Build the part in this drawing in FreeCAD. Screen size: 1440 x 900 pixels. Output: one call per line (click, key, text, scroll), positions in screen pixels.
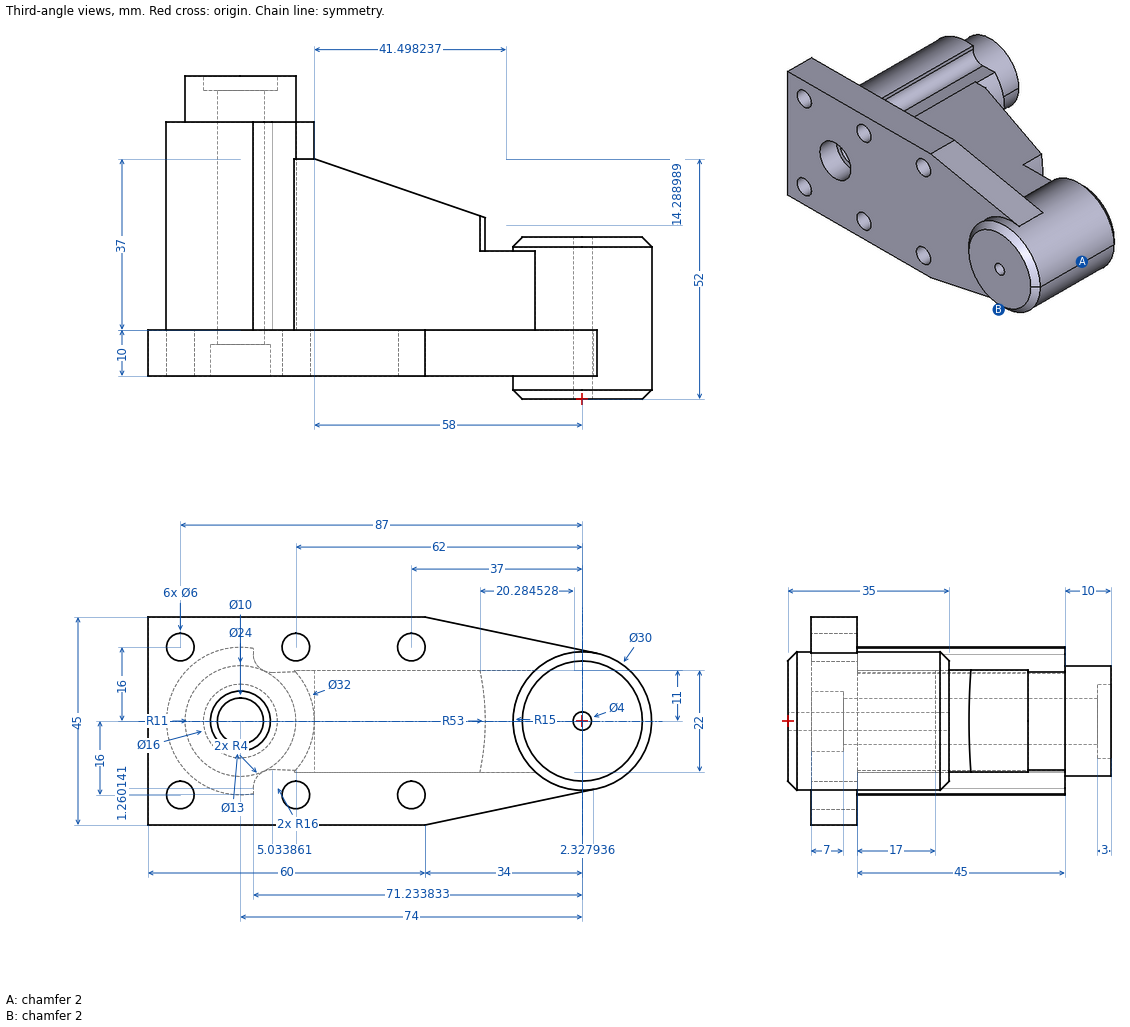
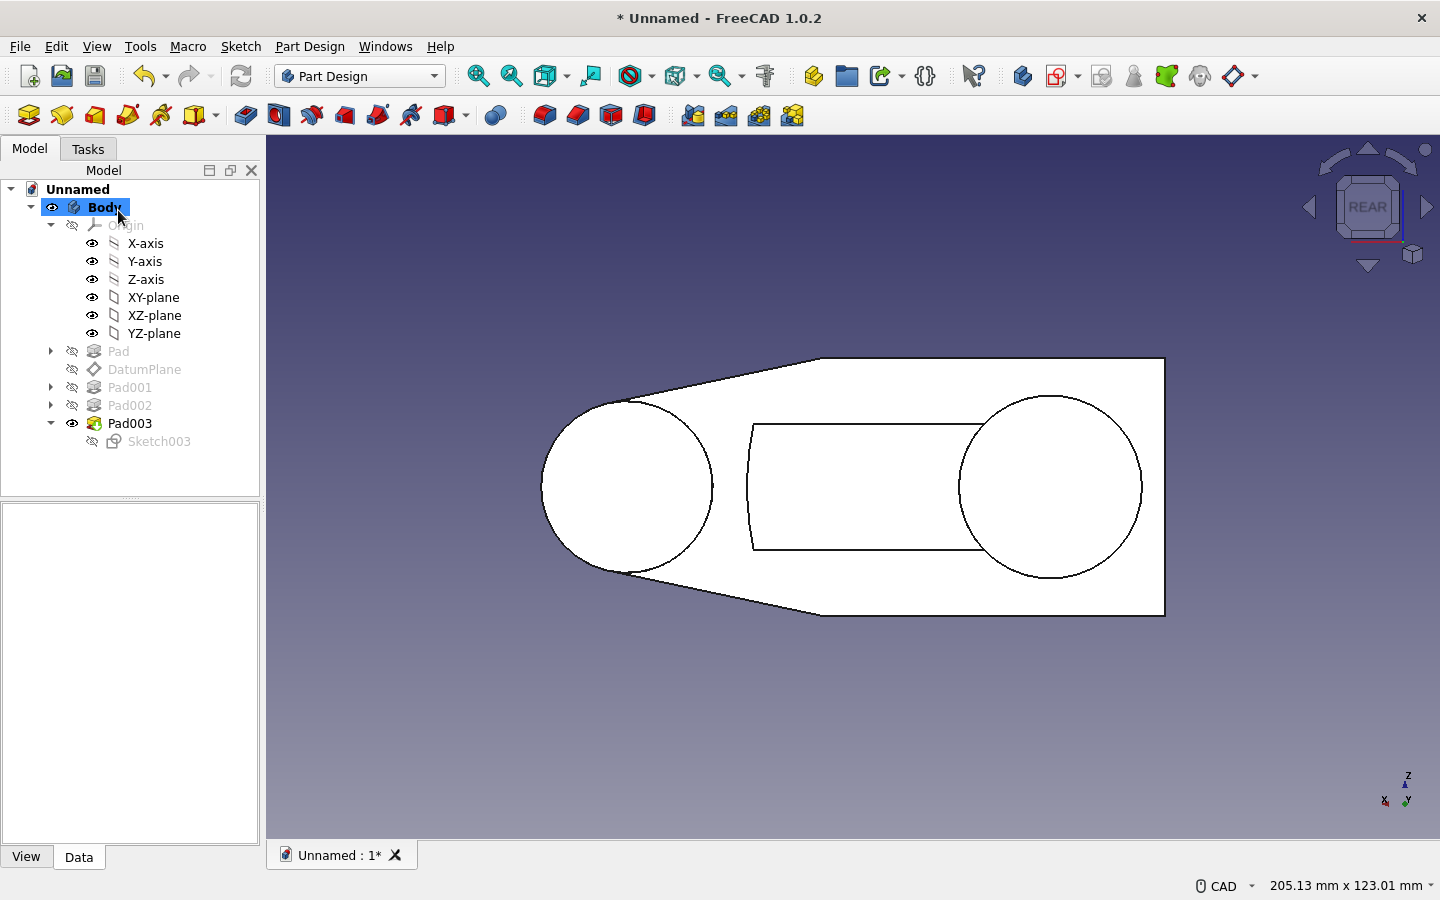
key(0)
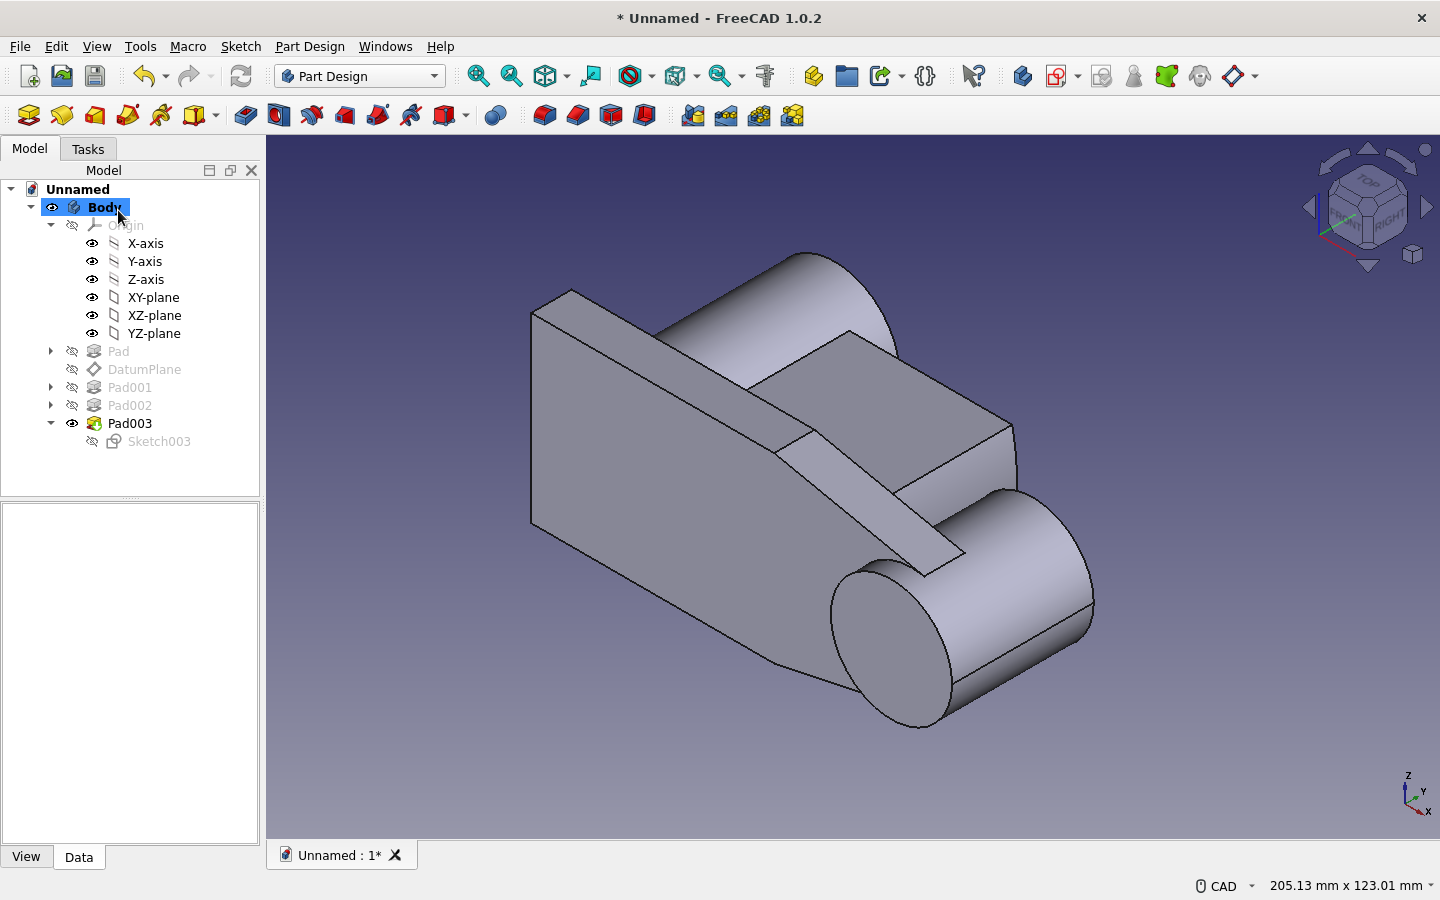
click(856, 420)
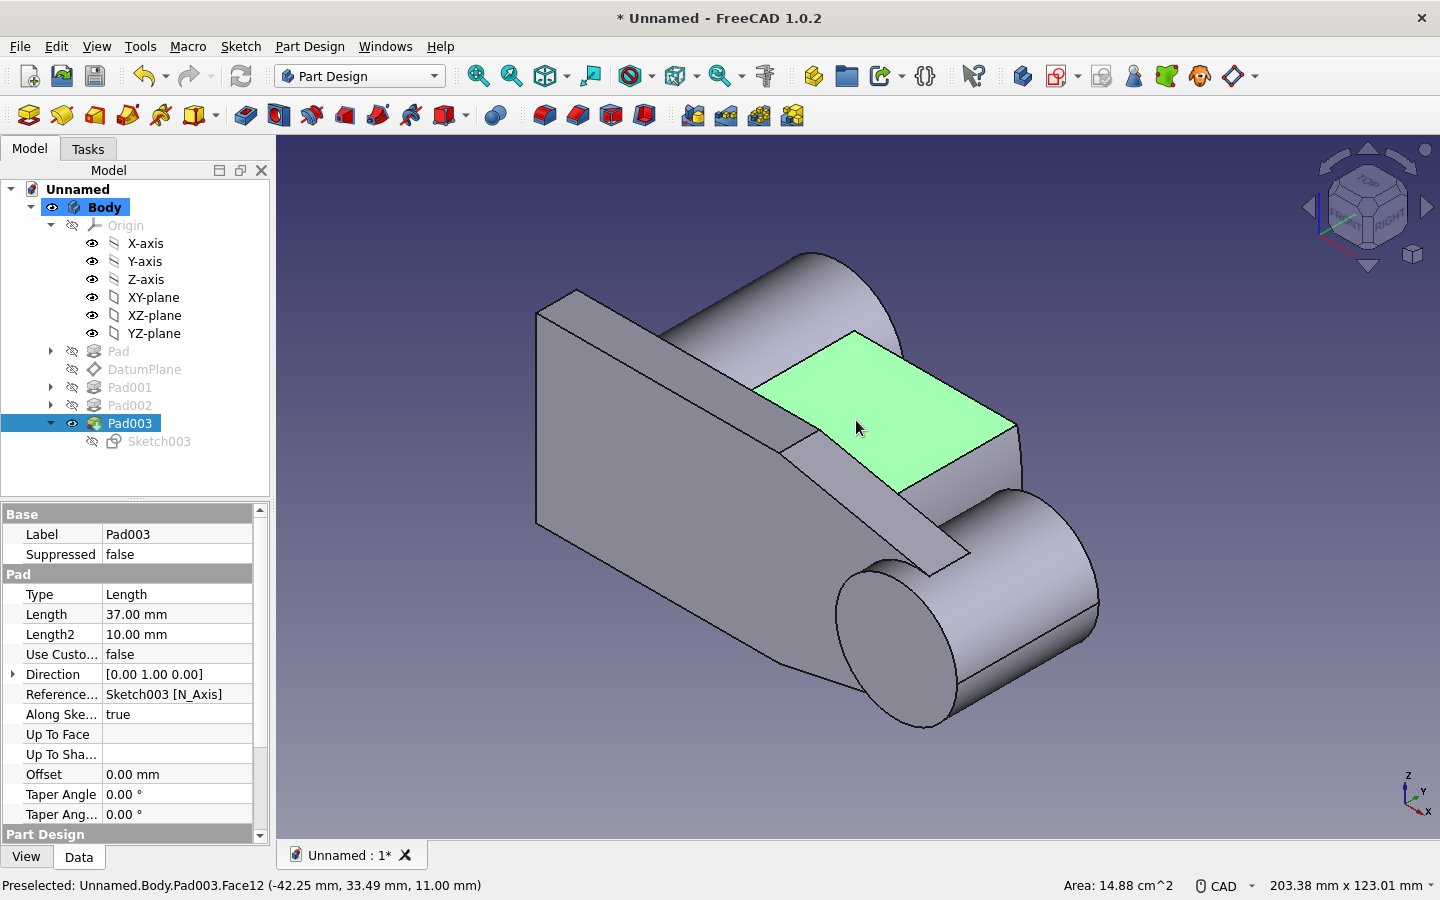
click(1056, 76)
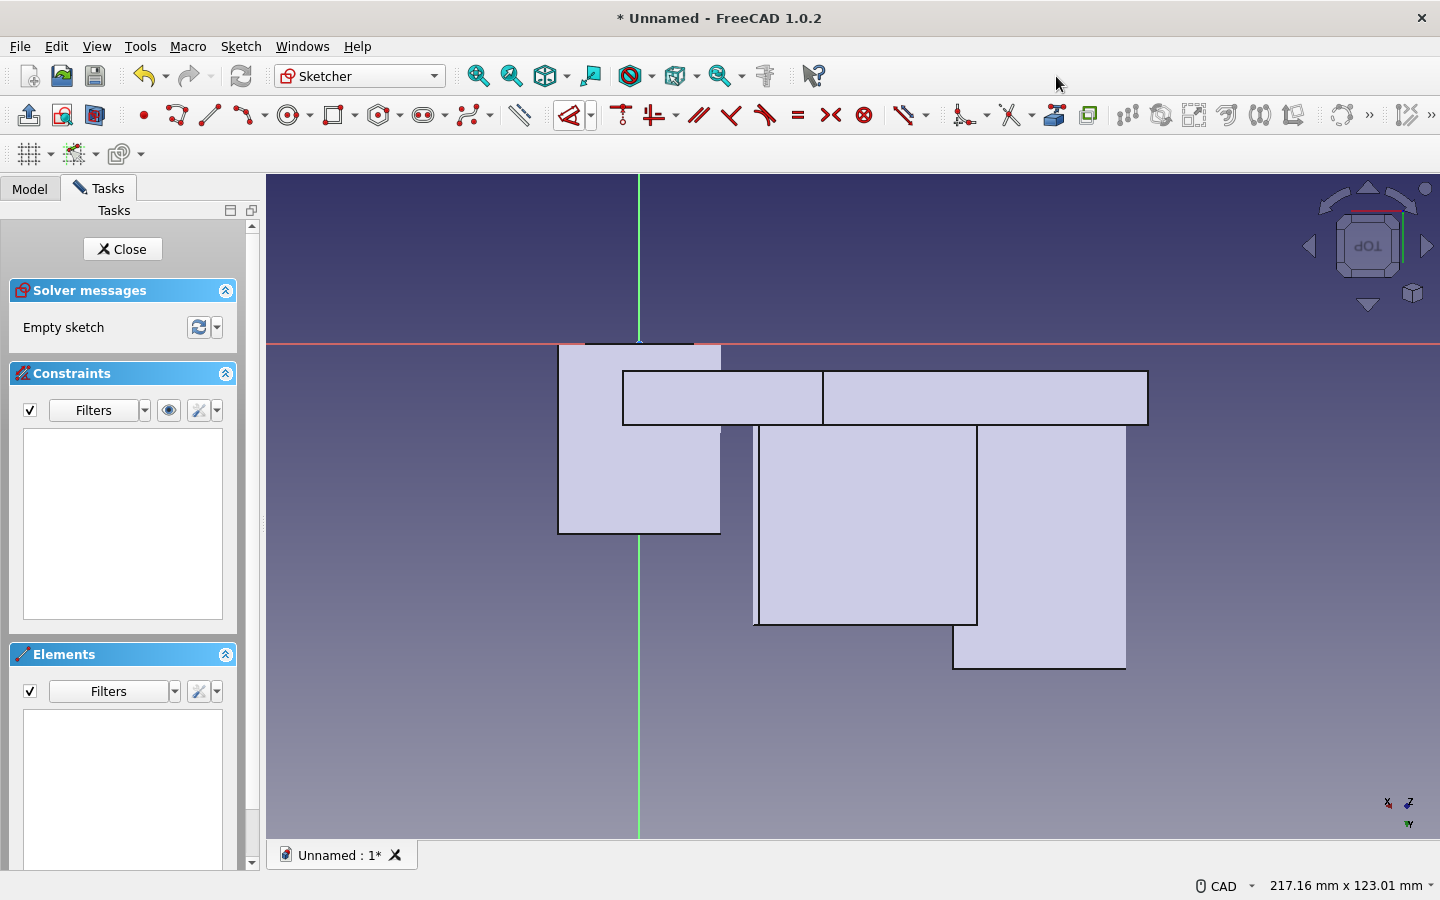
scroll(820, 441, up, 2)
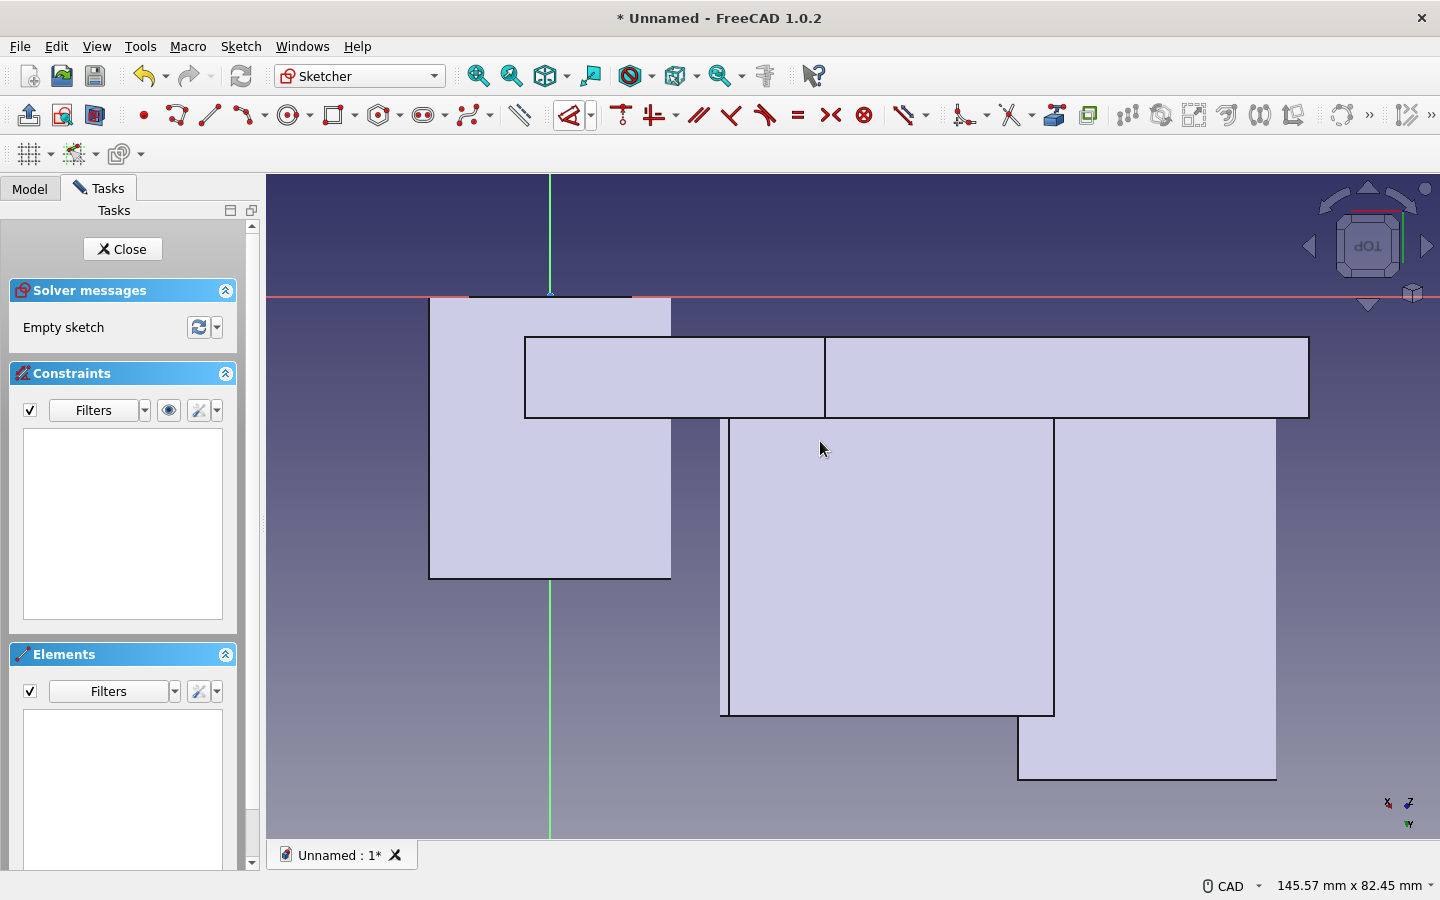
click(177, 116)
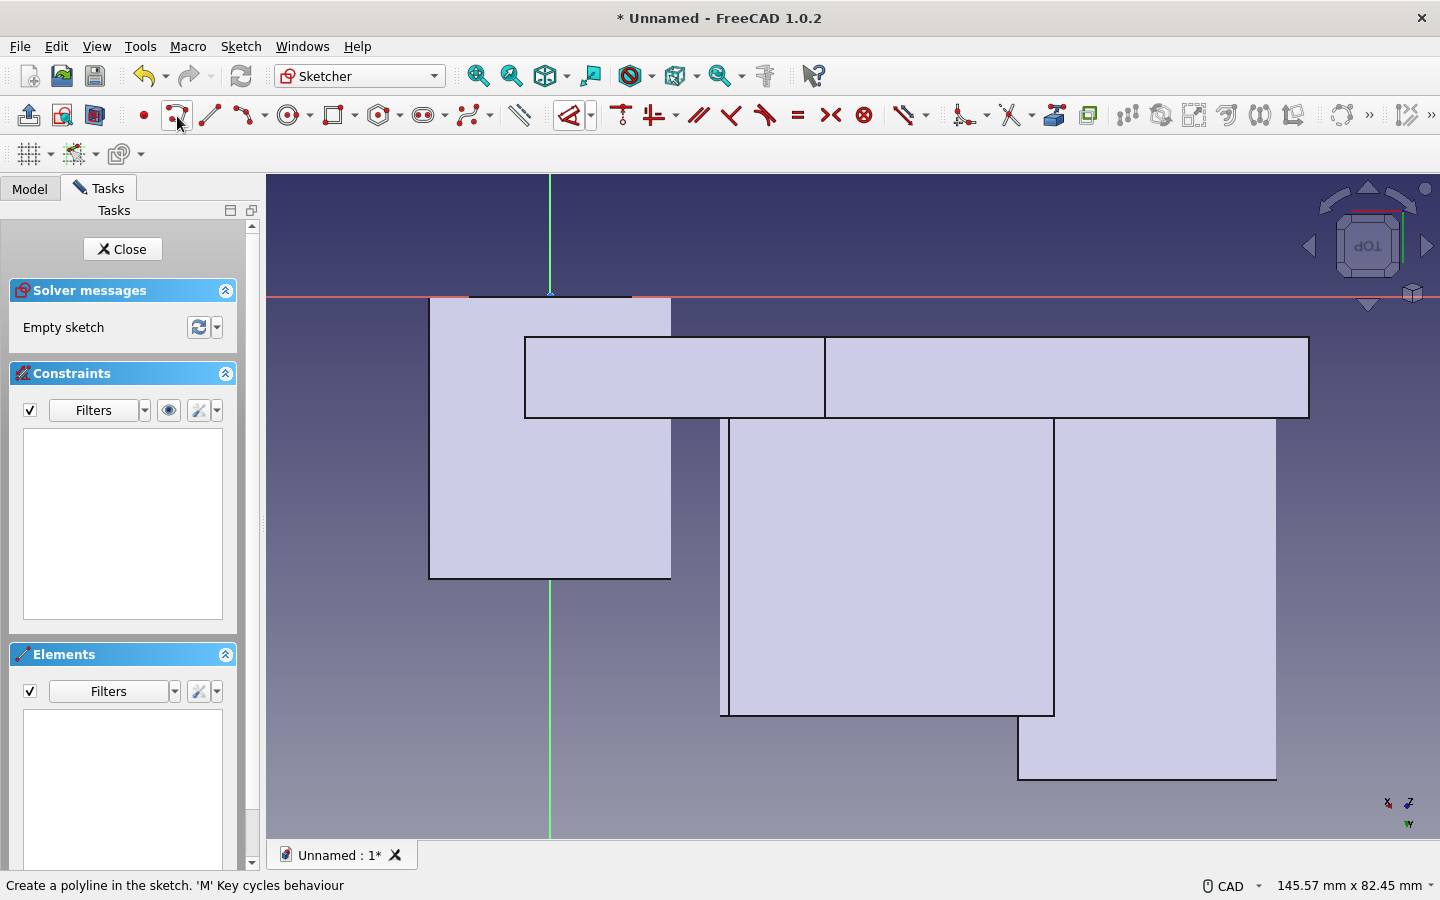
click(684, 601)
click(684, 716)
click(1018, 716)
click(684, 602)
key(Escape)
key(Escape)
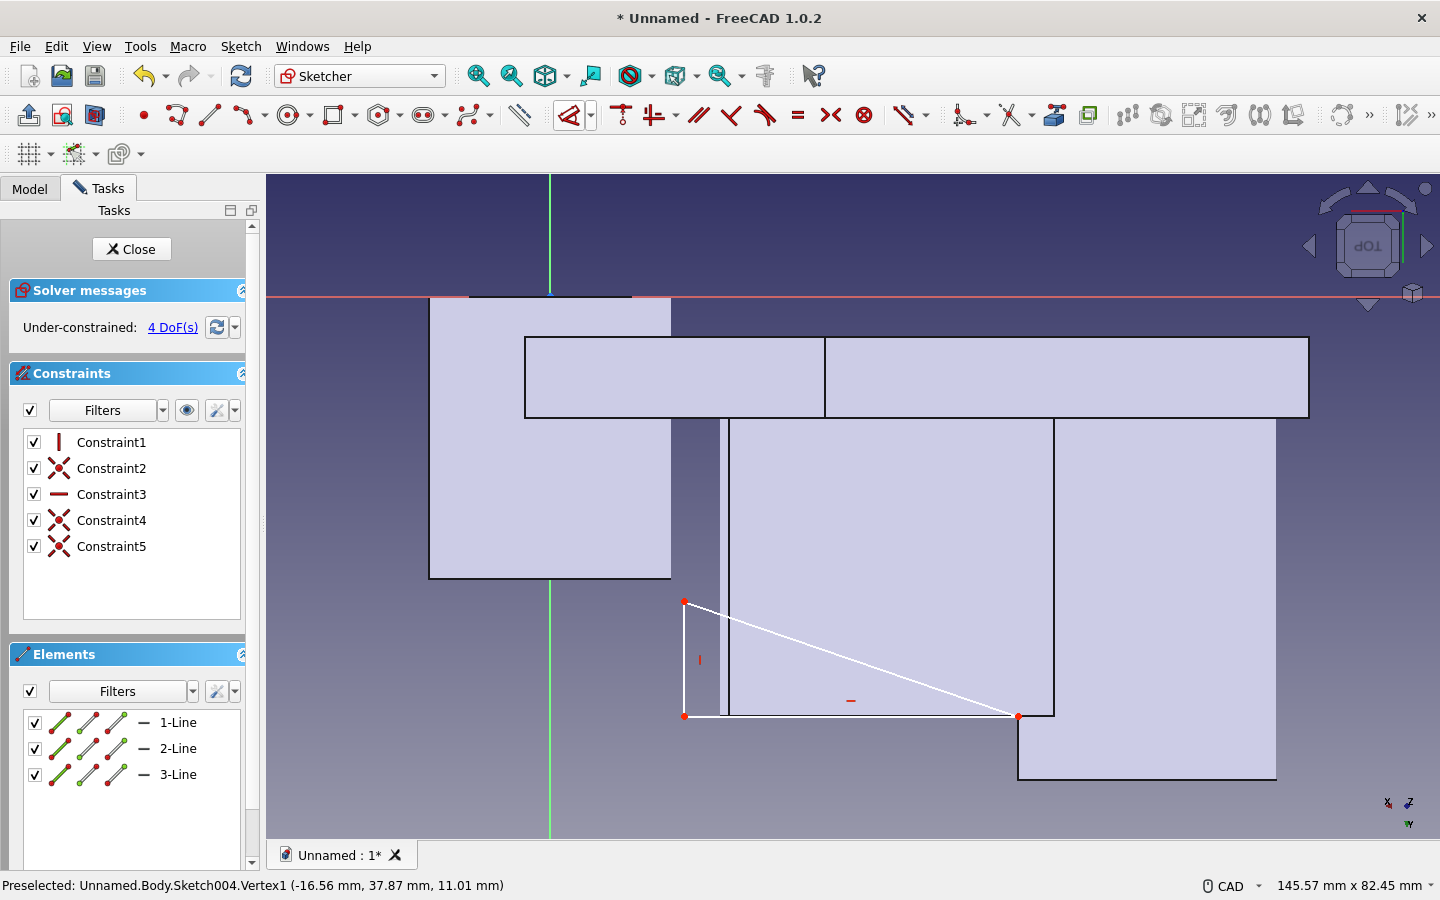
click(684, 717)